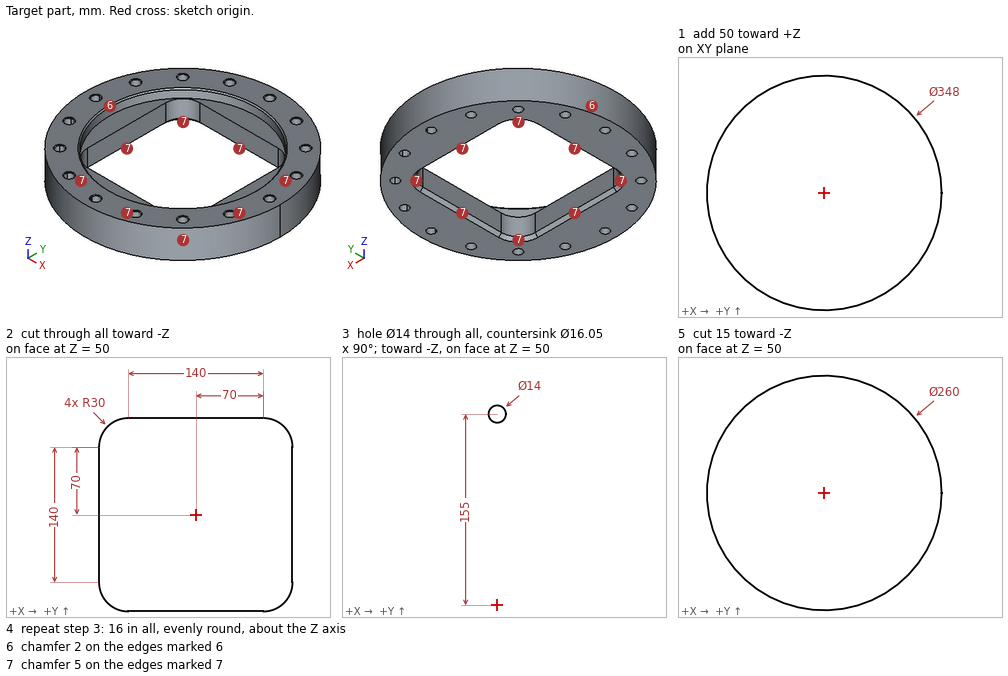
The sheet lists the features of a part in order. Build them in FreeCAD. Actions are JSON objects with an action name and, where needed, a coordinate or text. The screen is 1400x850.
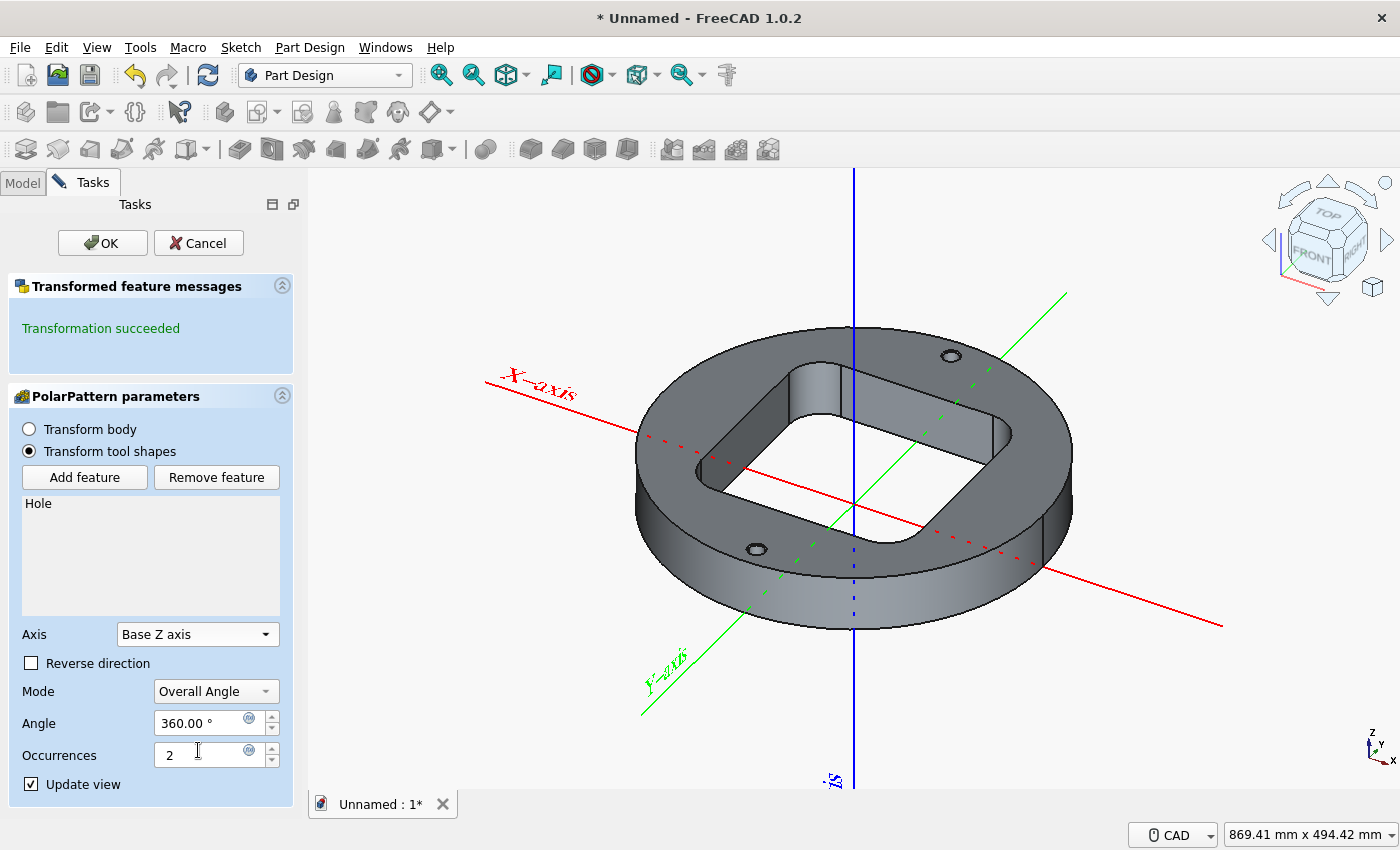
{"action": "triple_click", "coordinate": [209, 755]}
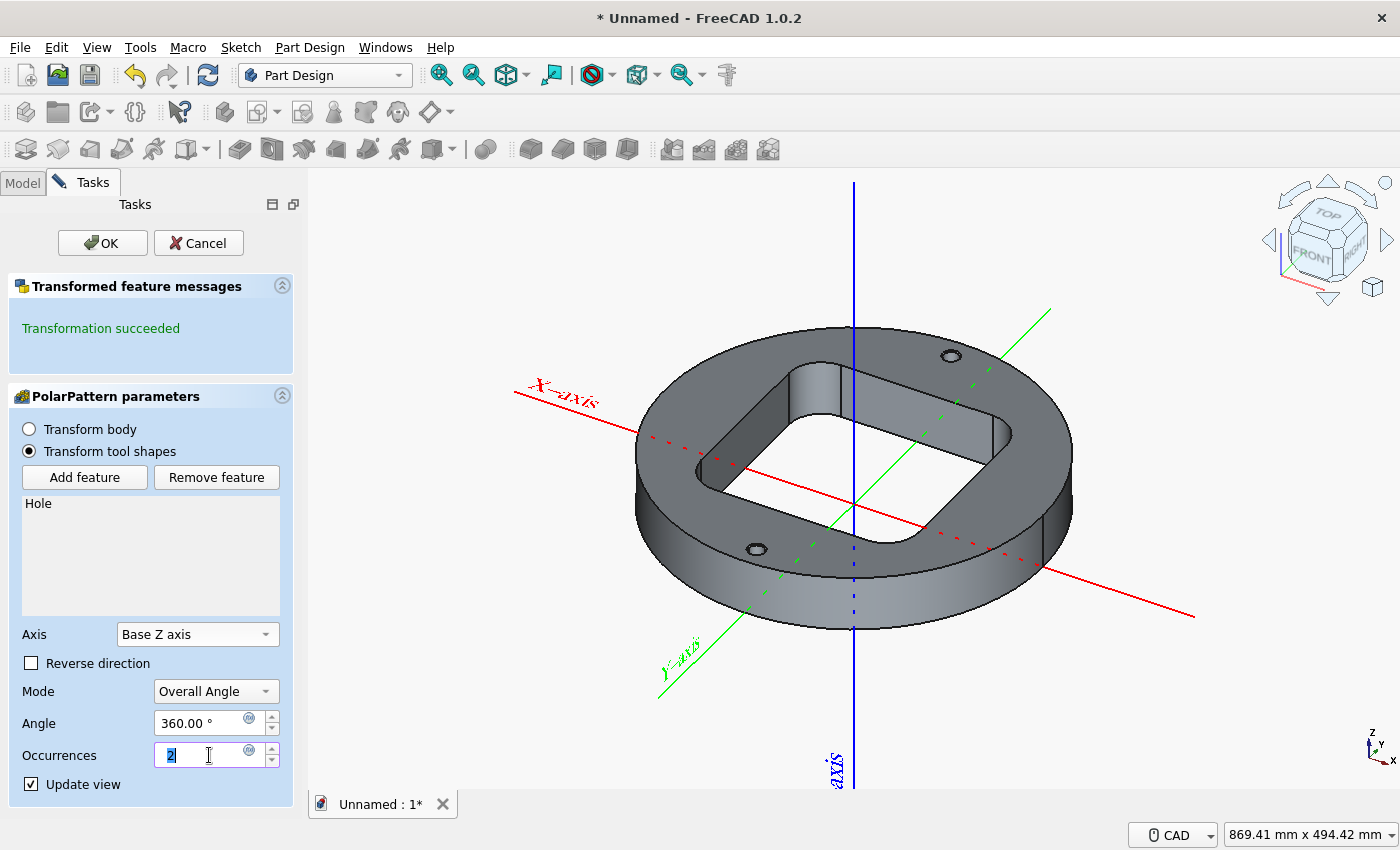
{"action": "type", "text": "16"}
{"action": "key", "text": "Tab"}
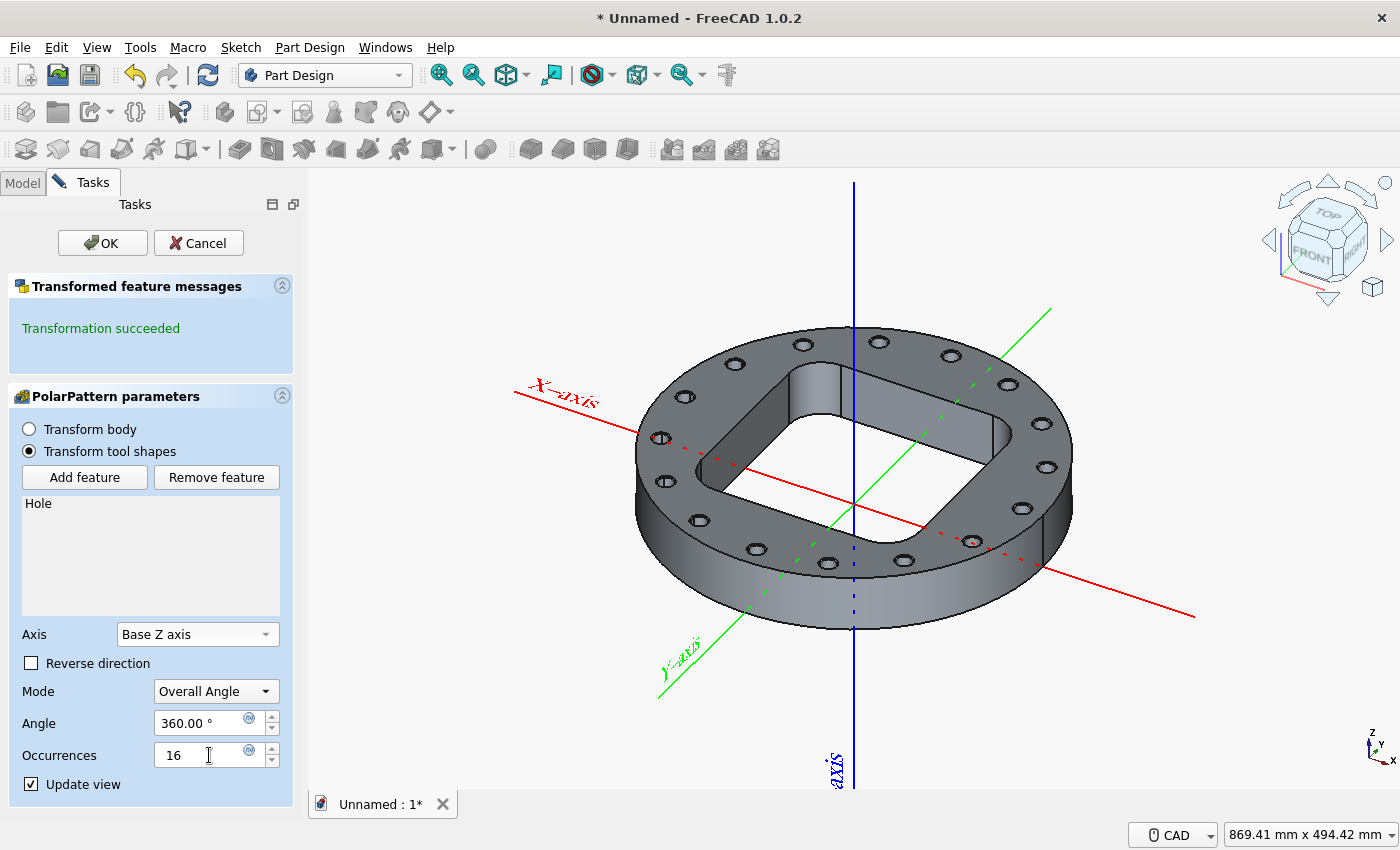
{"action": "left_click", "coordinate": [103, 243]}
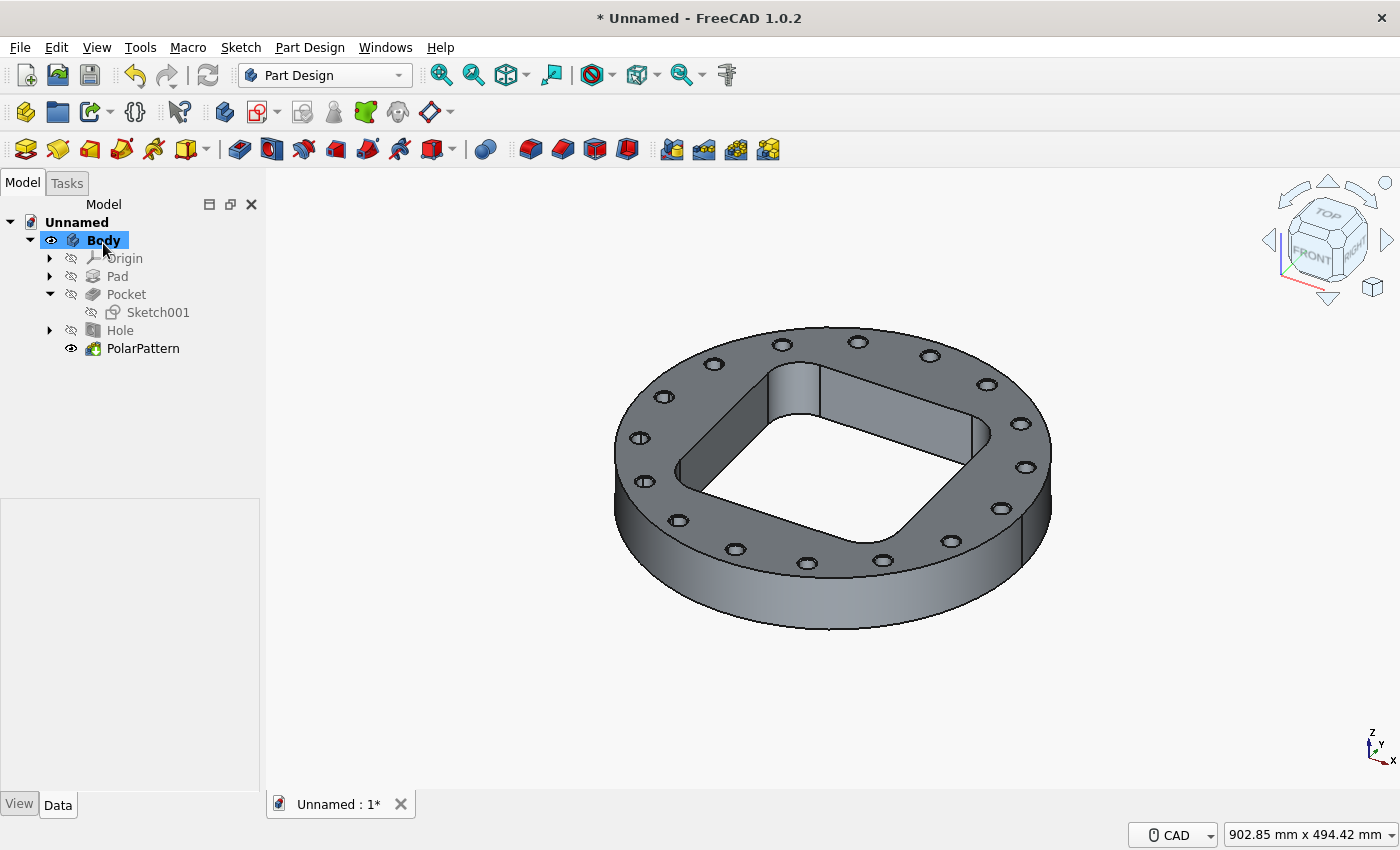
{"action": "left_click", "coordinate": [1003, 426]}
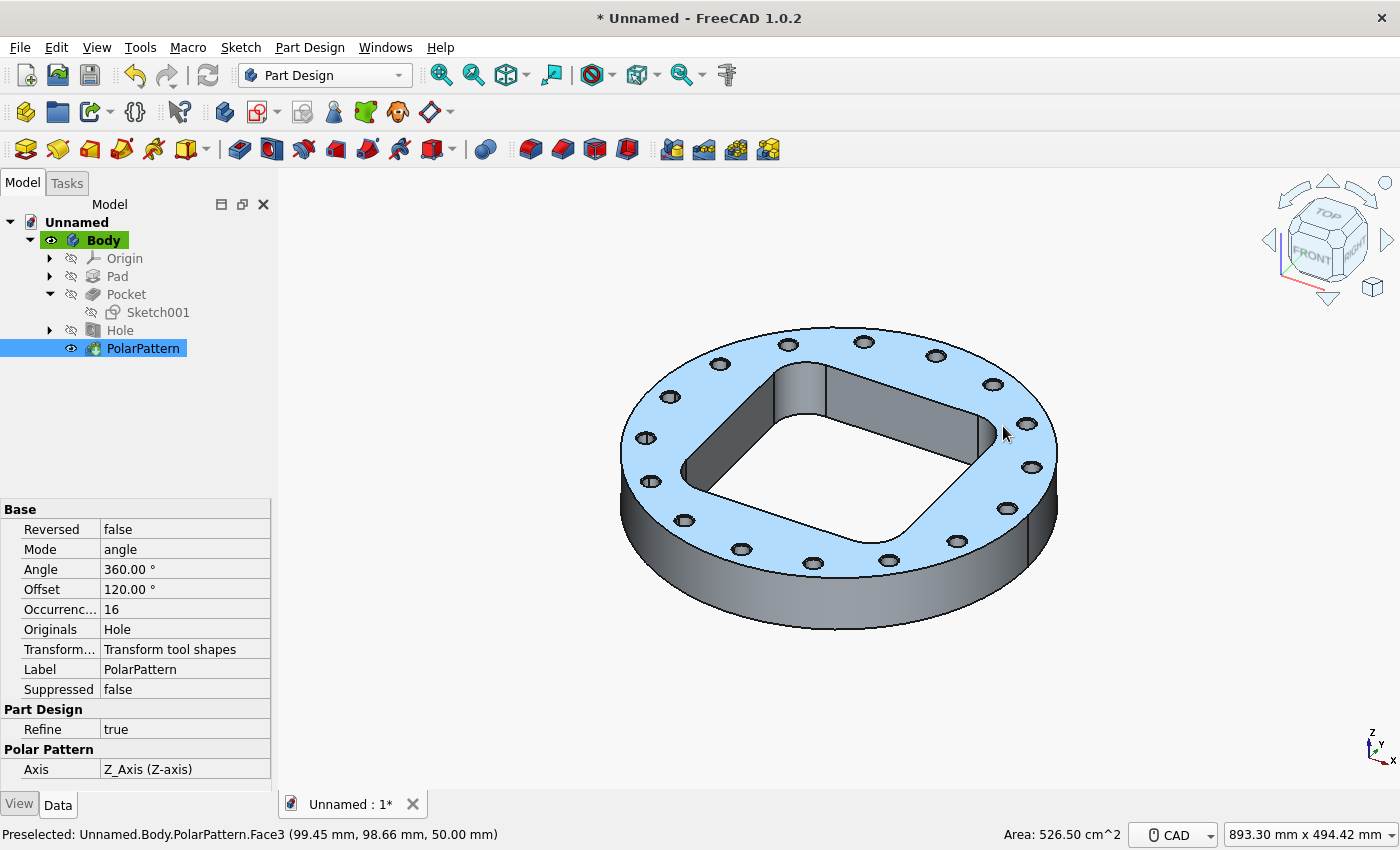
{"action": "left_click", "coordinate": [258, 112]}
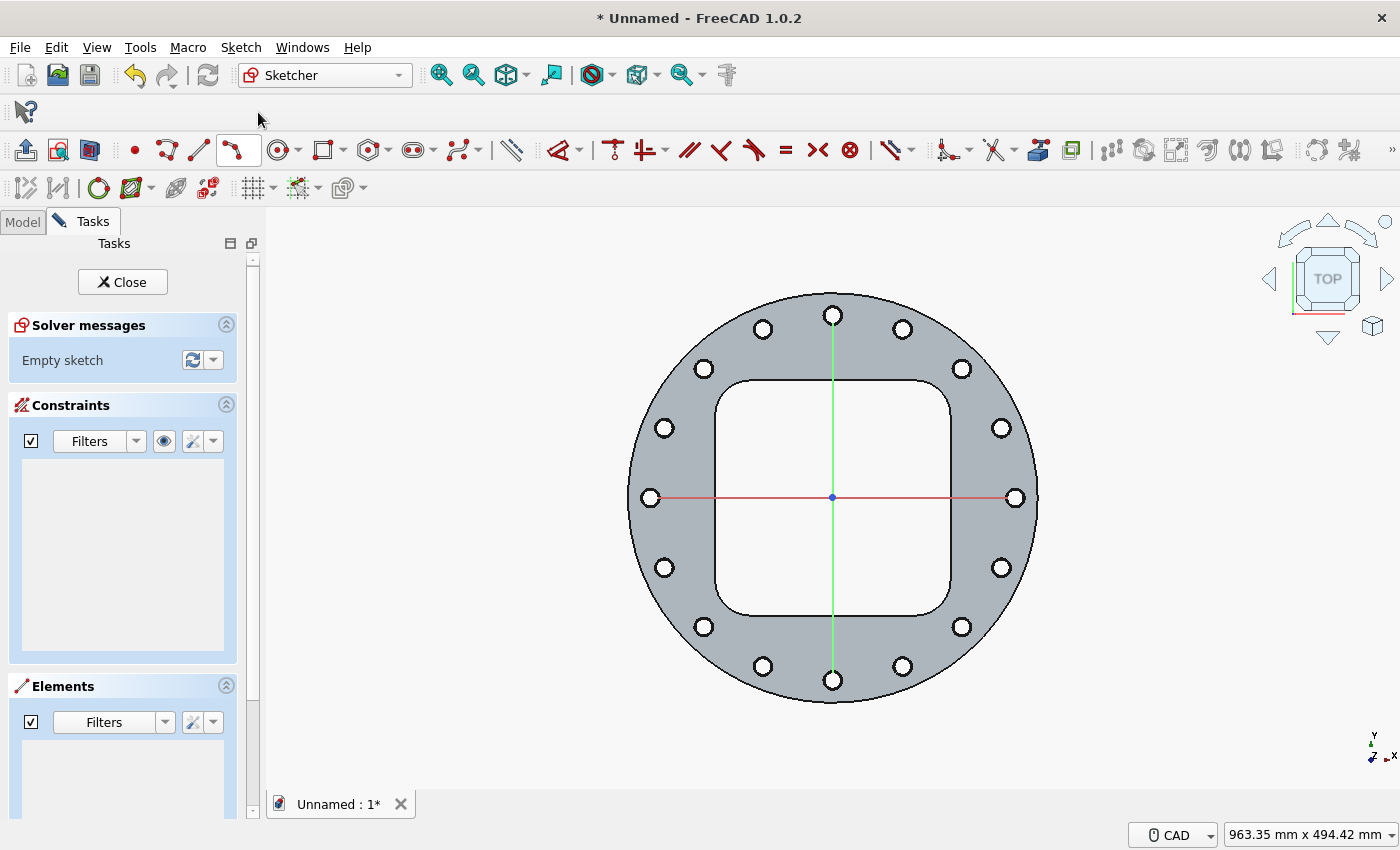
{"action": "left_click", "coordinate": [278, 150]}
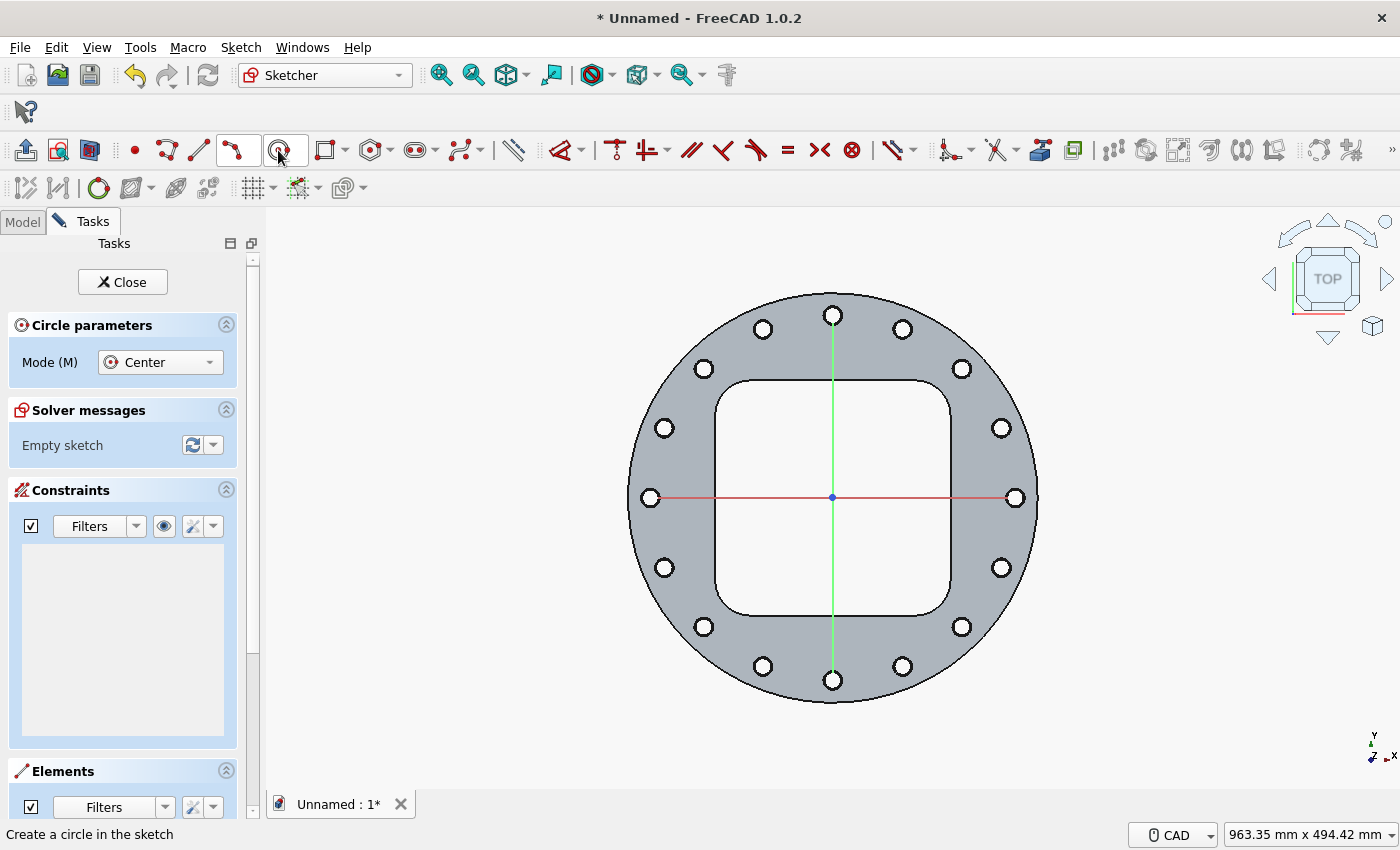
{"action": "left_click", "coordinate": [833, 498]}
{"action": "left_click", "coordinate": [941, 390]}
{"action": "key", "text": "Escape"}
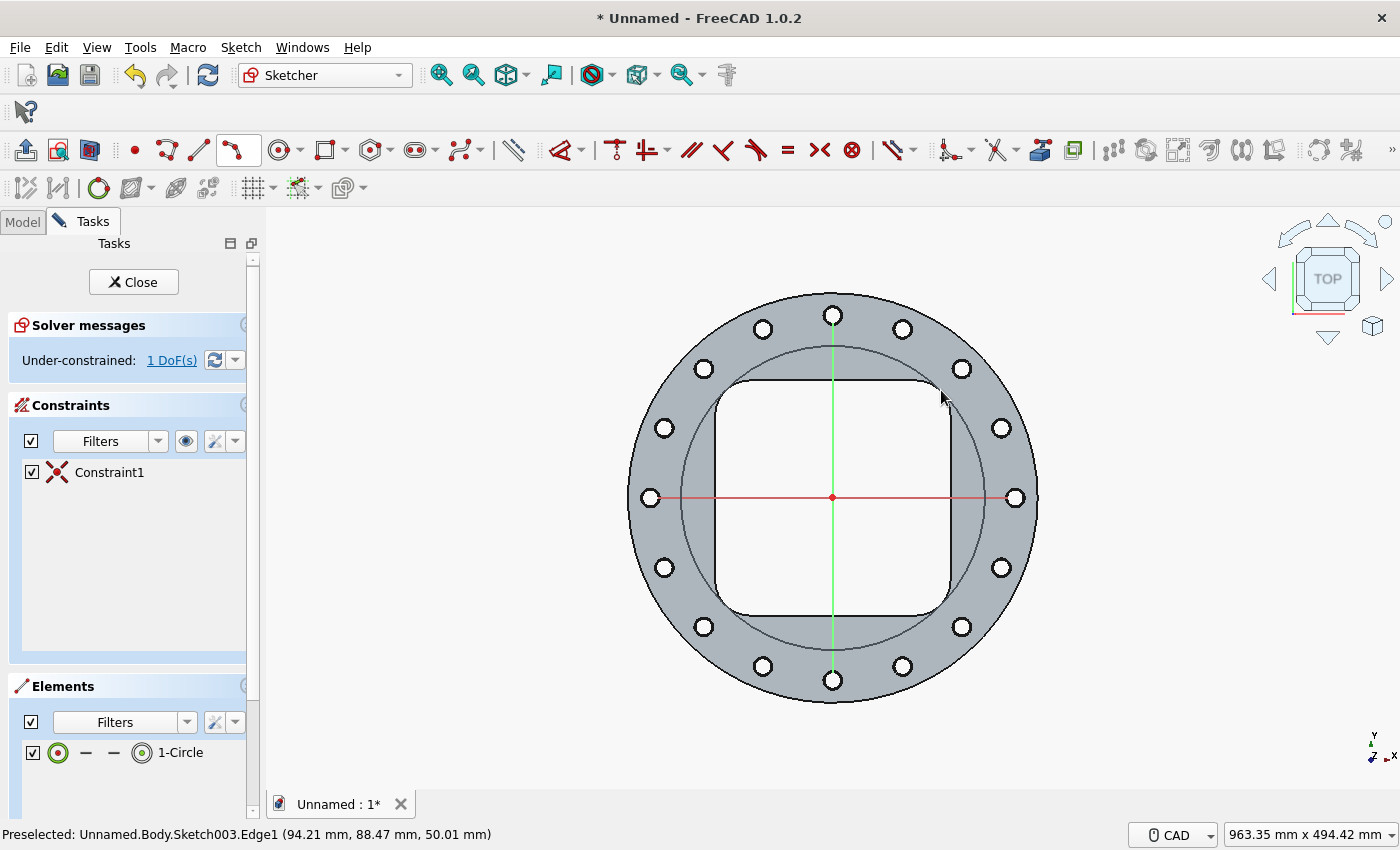
{"action": "left_click", "coordinate": [560, 150]}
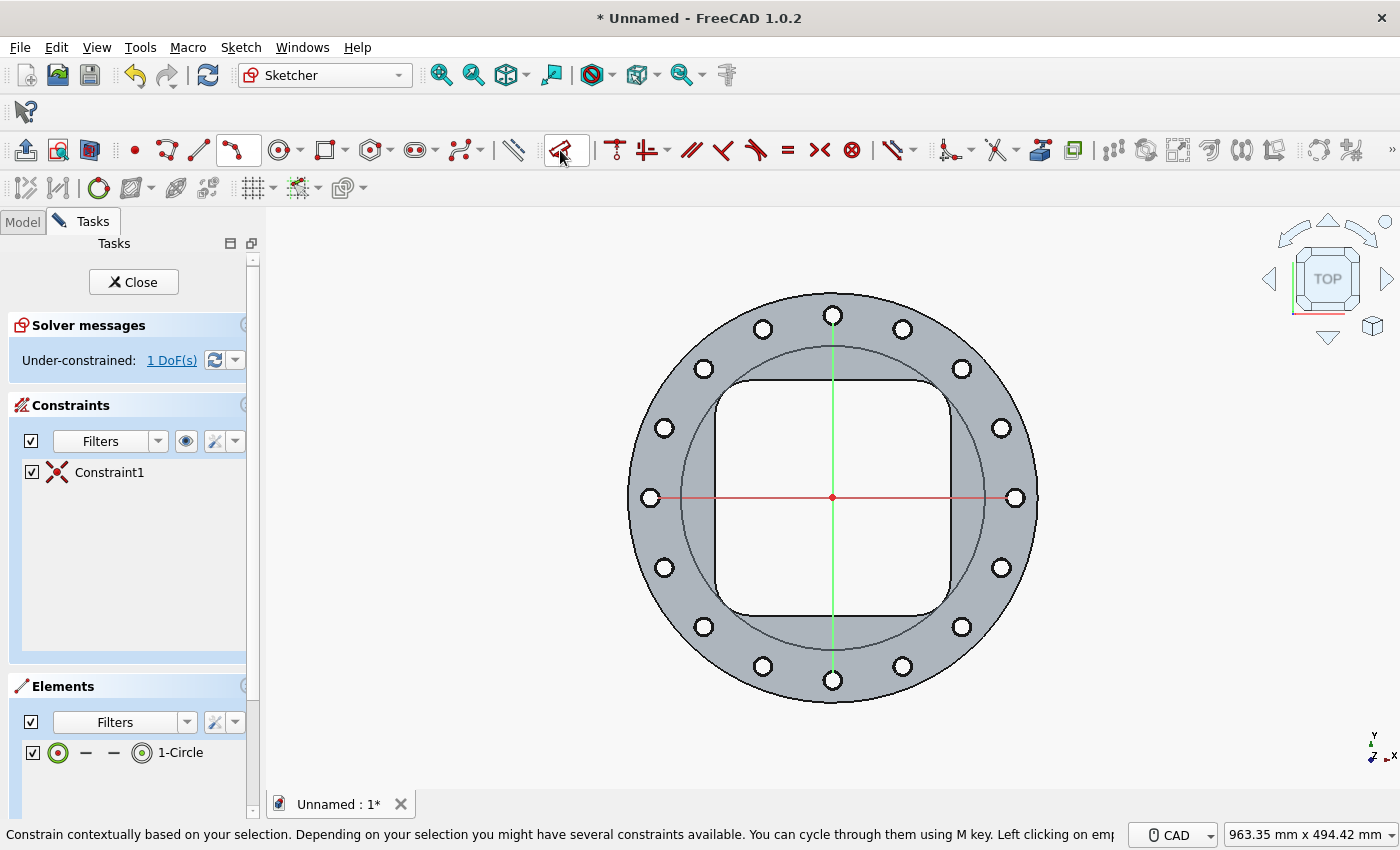
{"action": "left_click", "coordinate": [940, 390]}
{"action": "left_click", "coordinate": [963, 367]}